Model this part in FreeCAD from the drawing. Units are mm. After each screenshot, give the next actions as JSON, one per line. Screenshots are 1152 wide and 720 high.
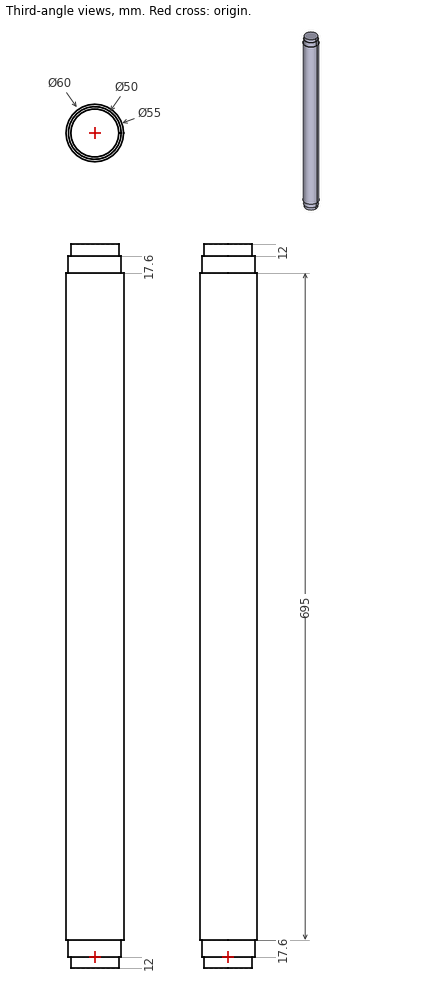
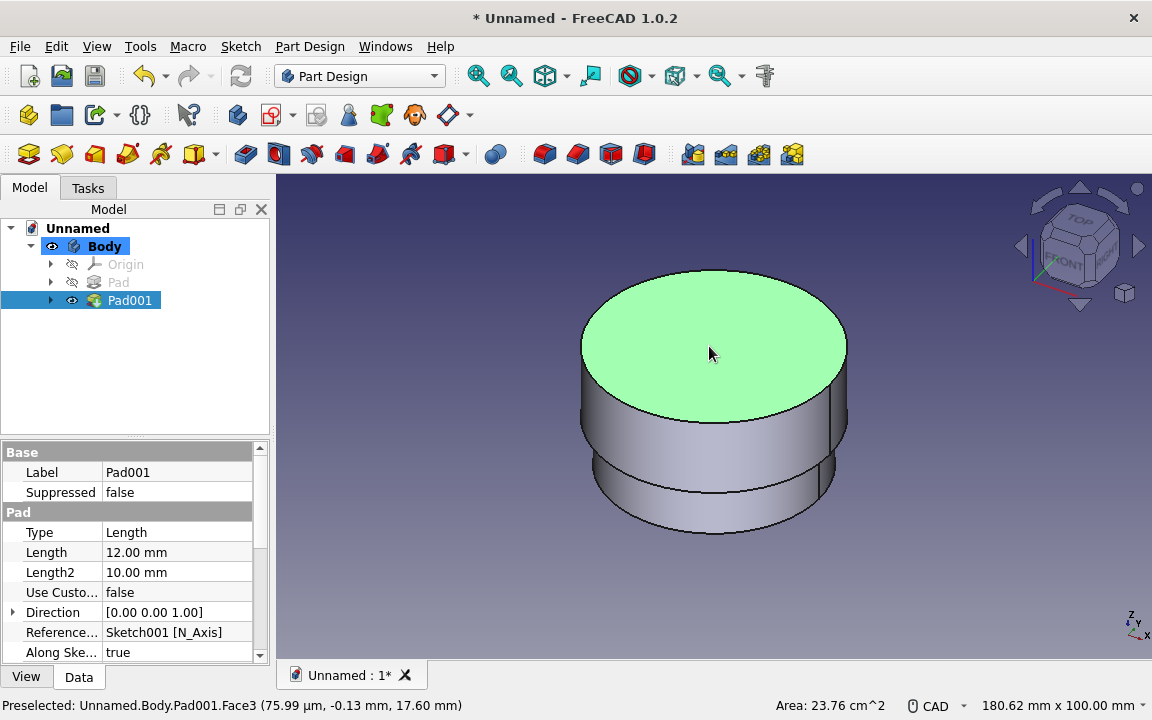
{"action": "left_click", "coordinate": [270, 116]}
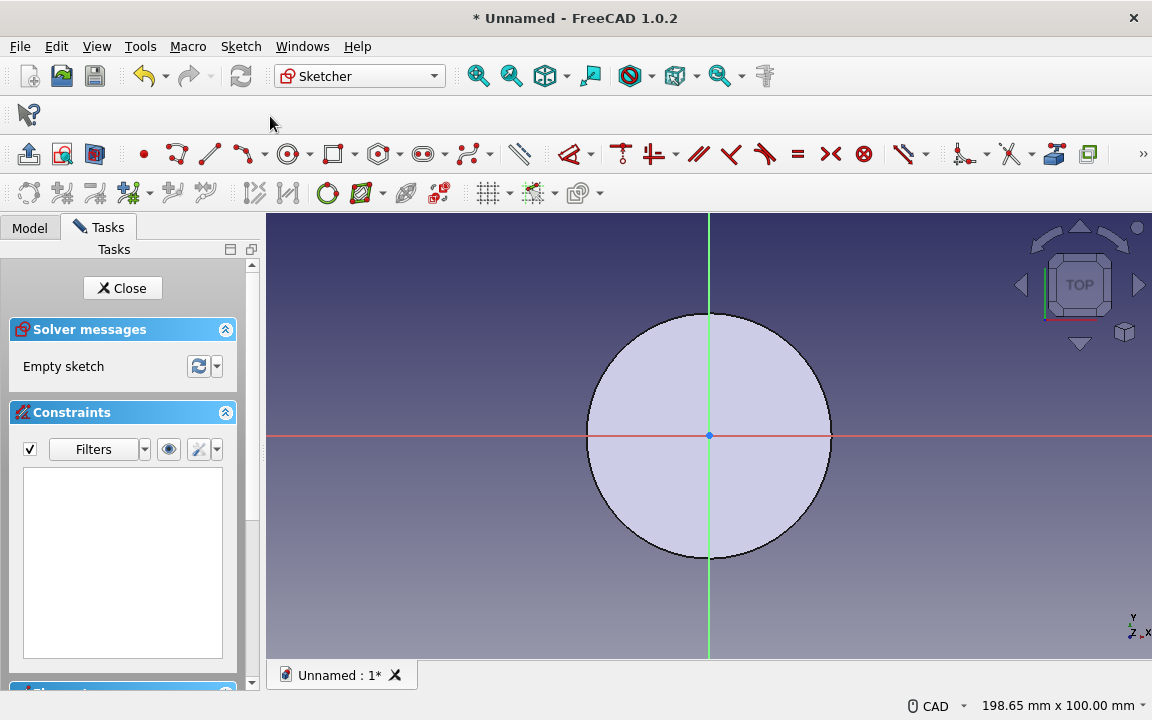
{"action": "left_click", "coordinate": [288, 154]}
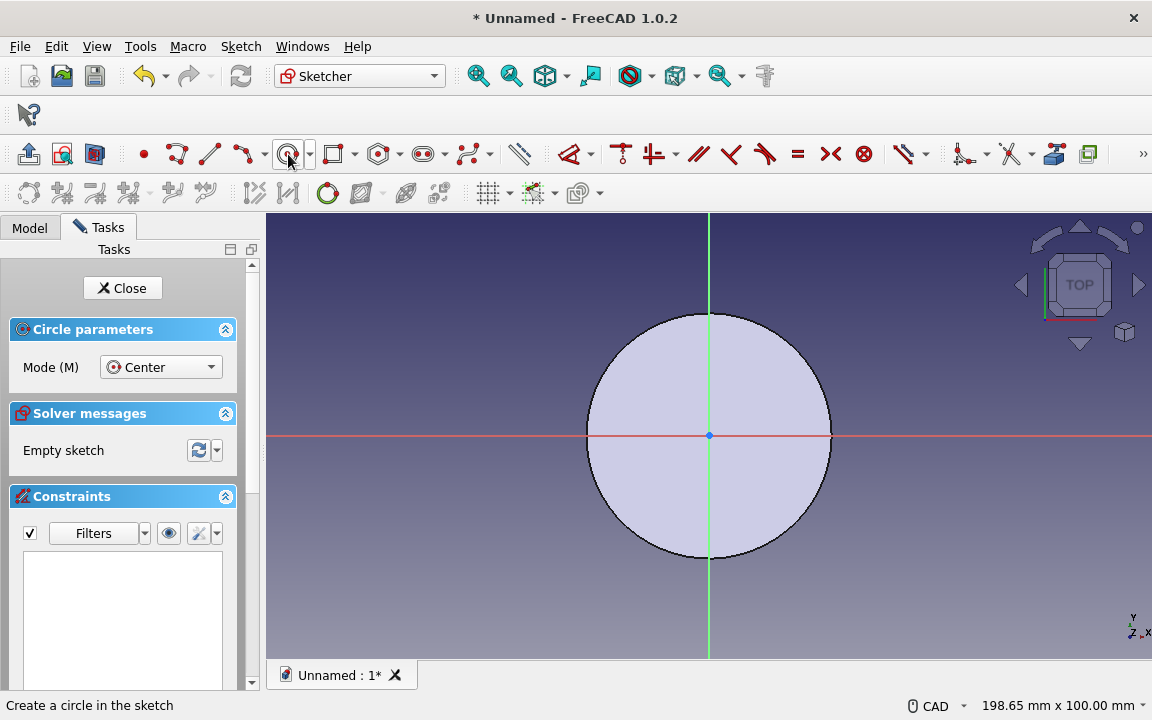
{"action": "left_click", "coordinate": [709, 436]}
{"action": "mouse_move", "coordinate": [804, 341]}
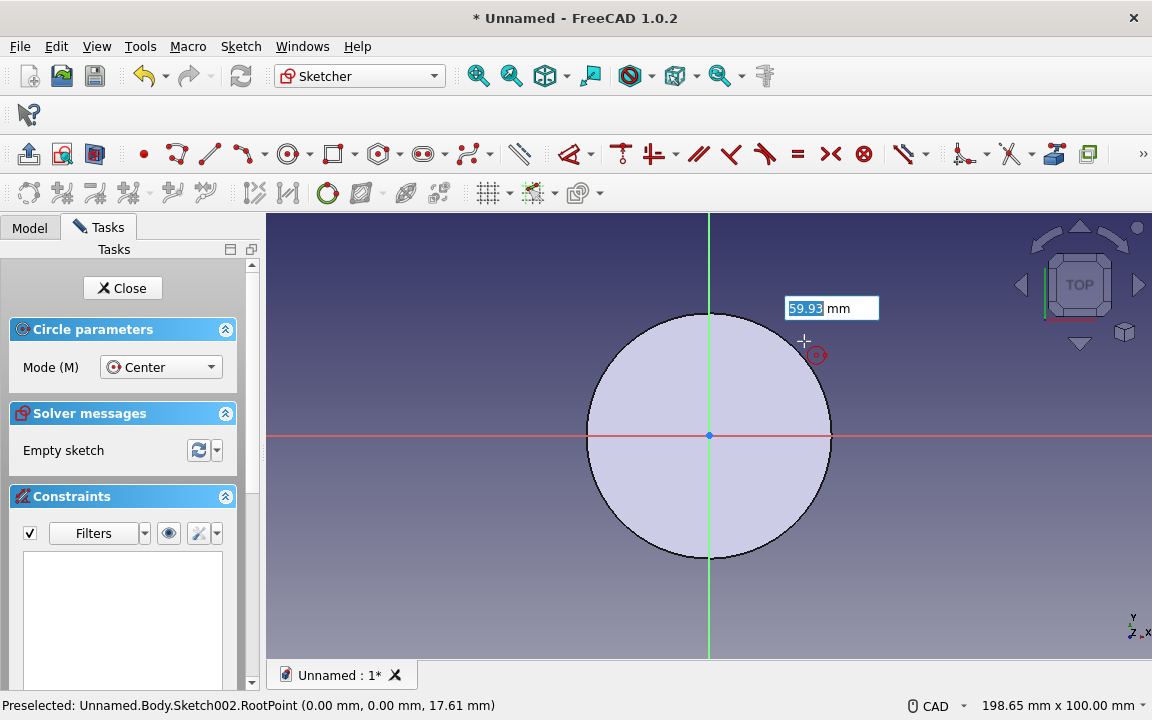
{"action": "type", "text": "60"}
{"action": "key", "text": "Return"}
{"action": "key", "text": "Escape"}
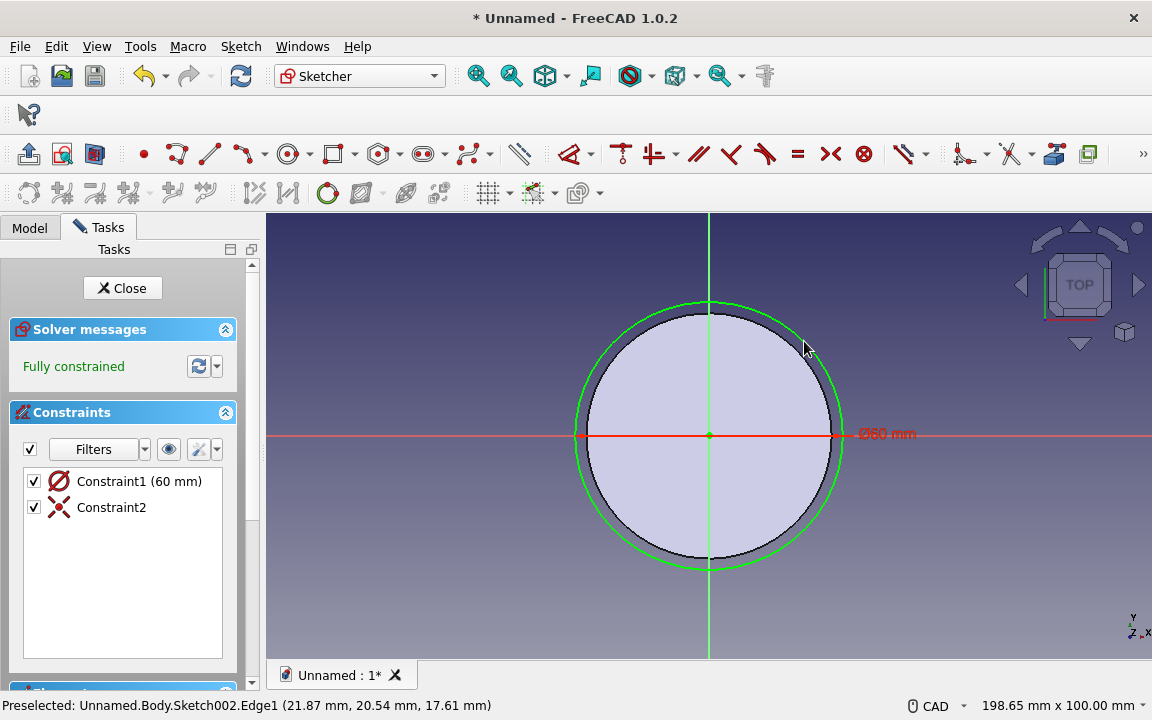
{"action": "left_click", "coordinate": [123, 288]}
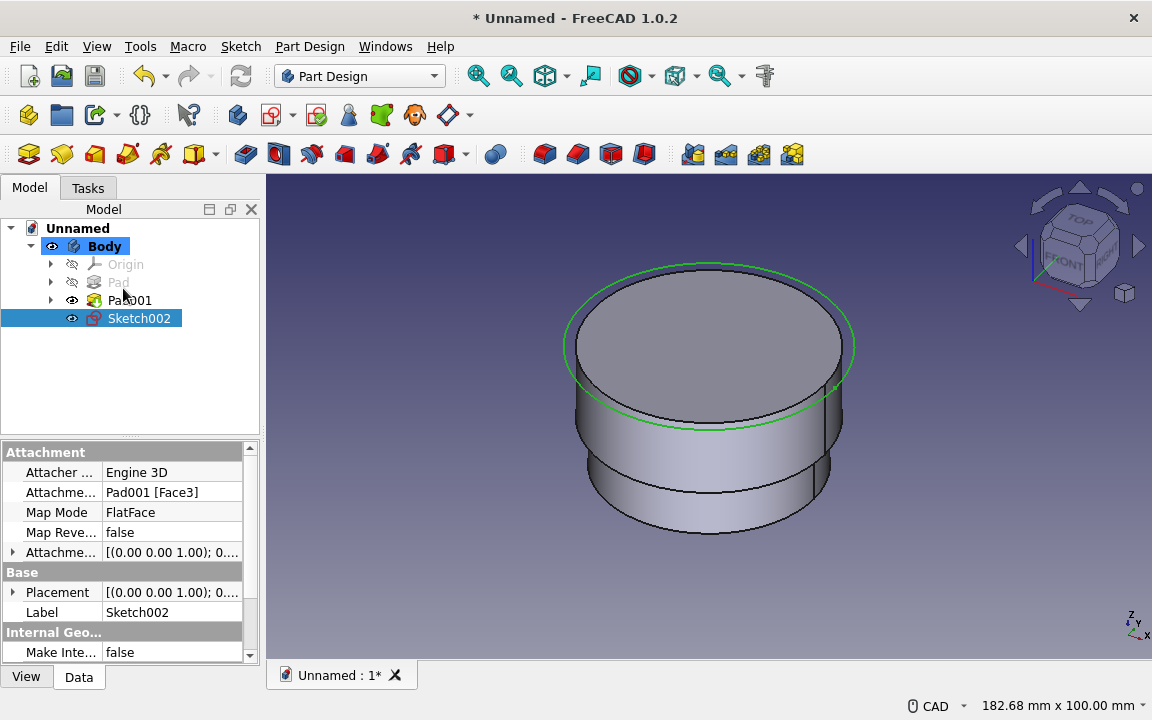
{"action": "left_click", "coordinate": [29, 154]}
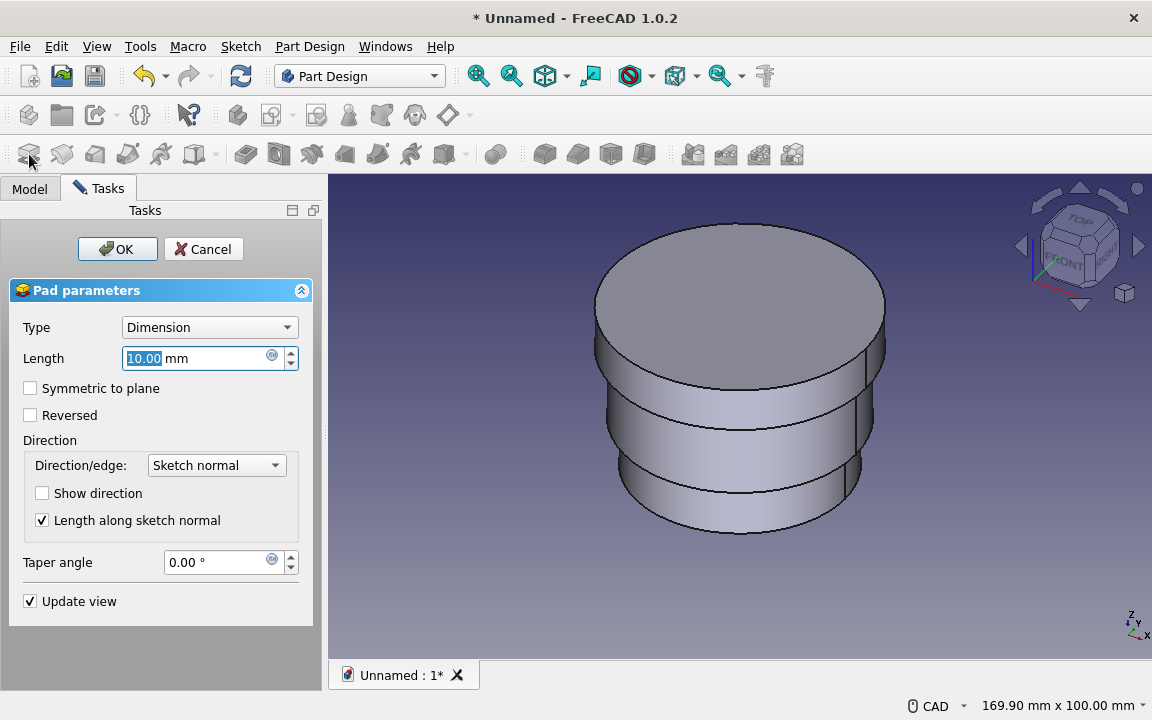
{"action": "type", "text": "695"}
{"action": "key", "text": "Tab"}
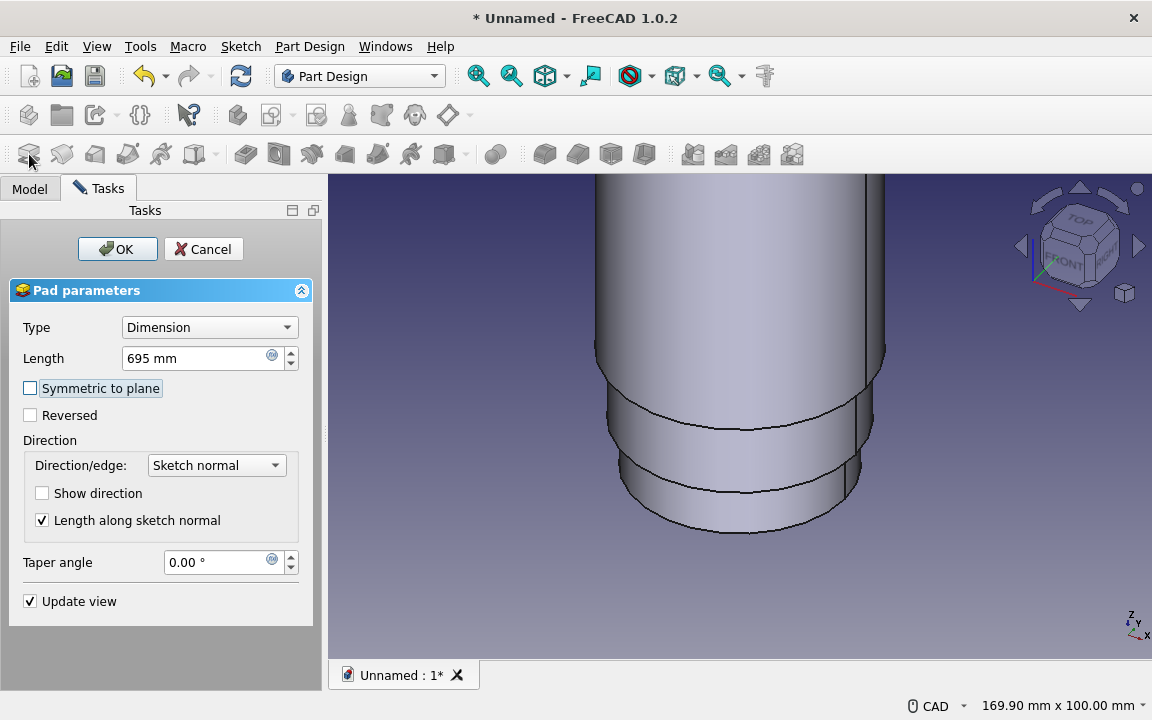
{"action": "left_click", "coordinate": [118, 249]}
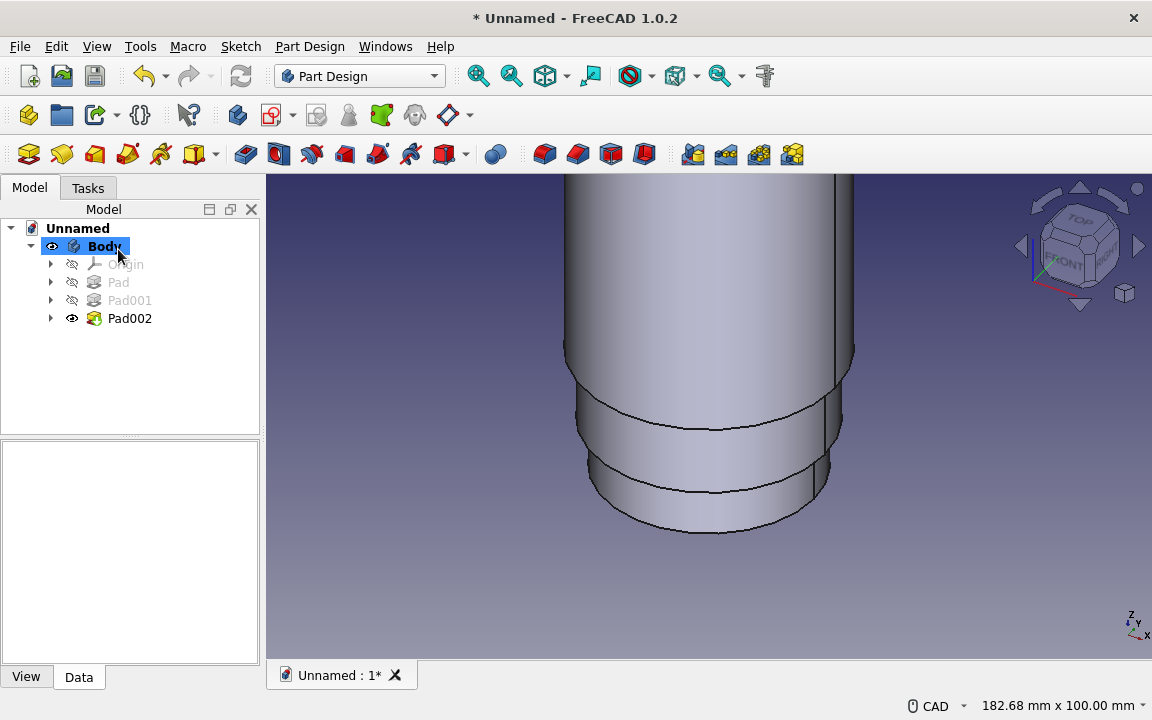
{"action": "key", "text": "v f"}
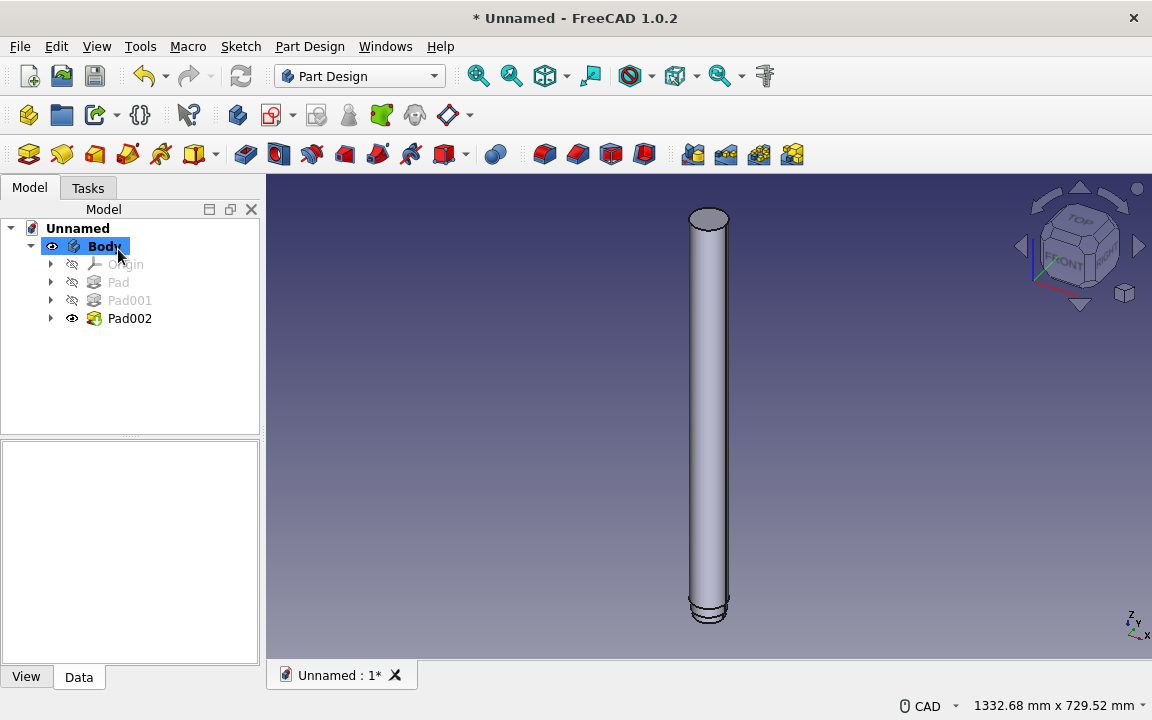
{"action": "left_click", "coordinate": [709, 218]}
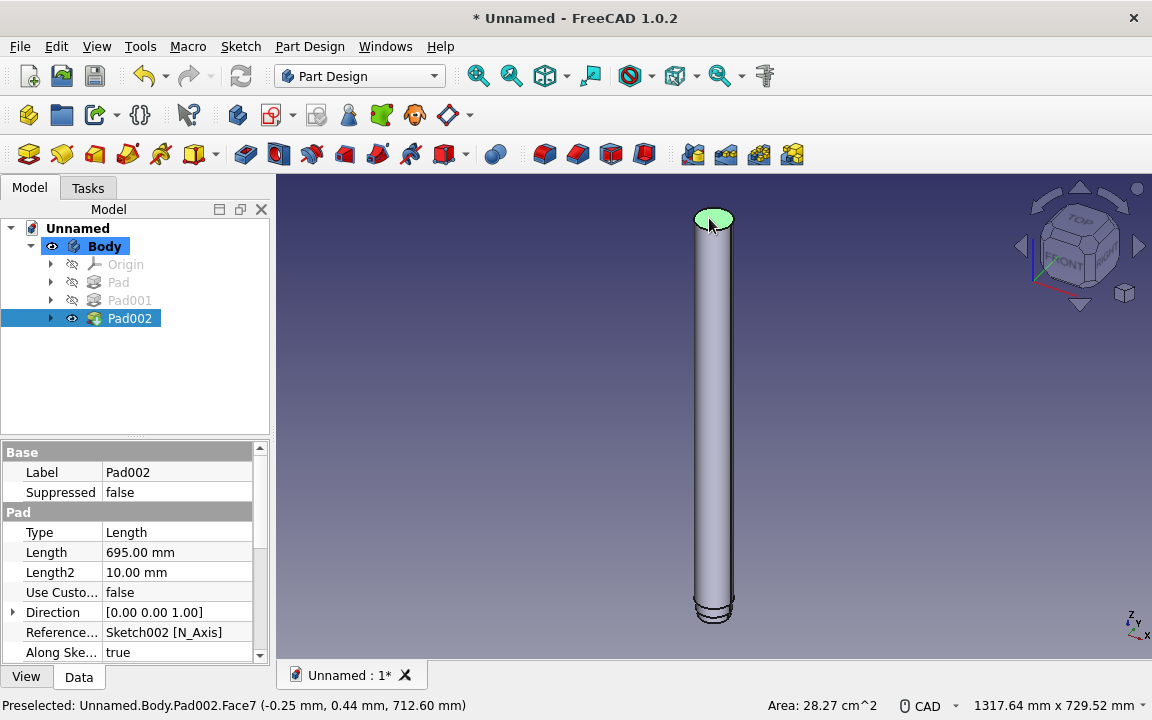
{"action": "left_click", "coordinate": [270, 116]}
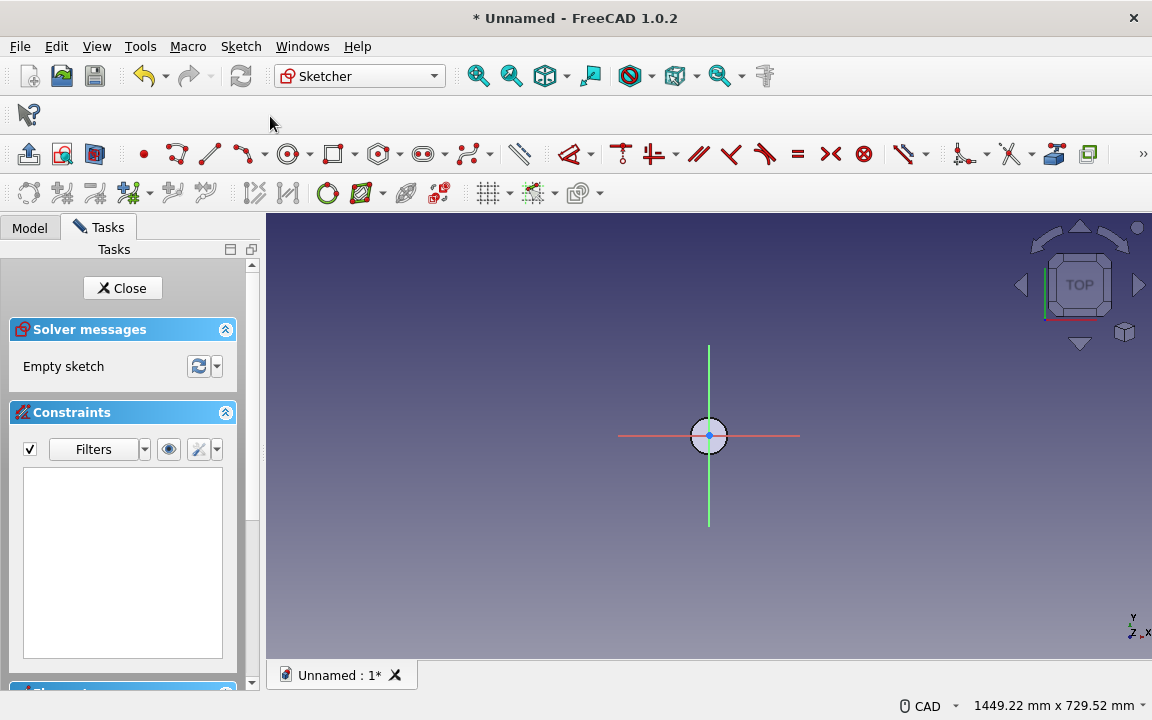
{"action": "scroll", "coordinate": [718, 436], "scroll_direction": "up", "scroll_amount": 11}